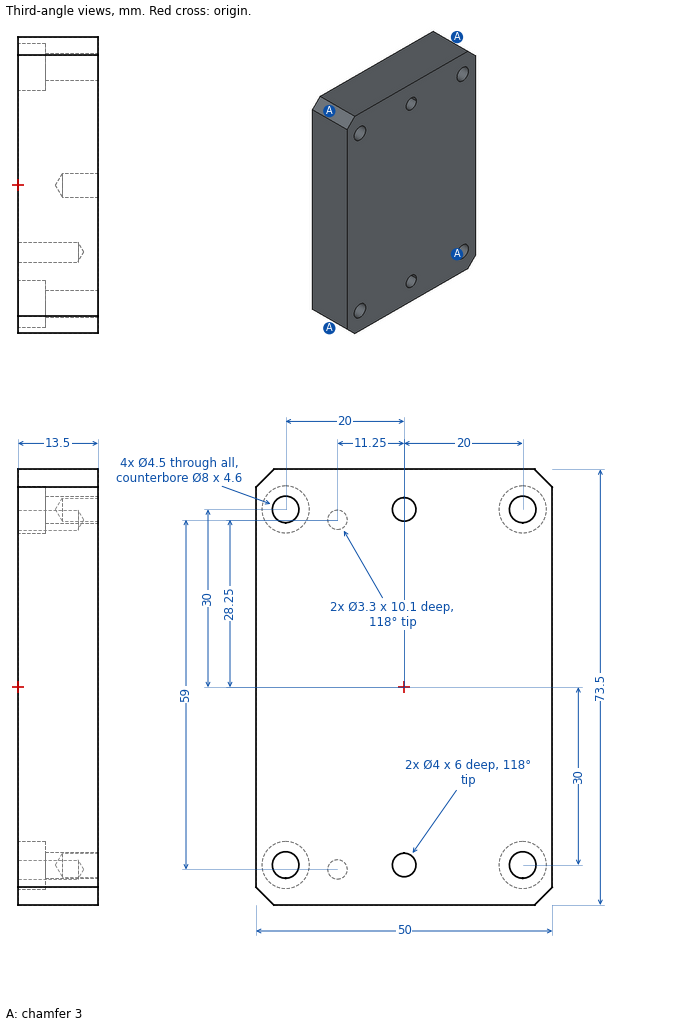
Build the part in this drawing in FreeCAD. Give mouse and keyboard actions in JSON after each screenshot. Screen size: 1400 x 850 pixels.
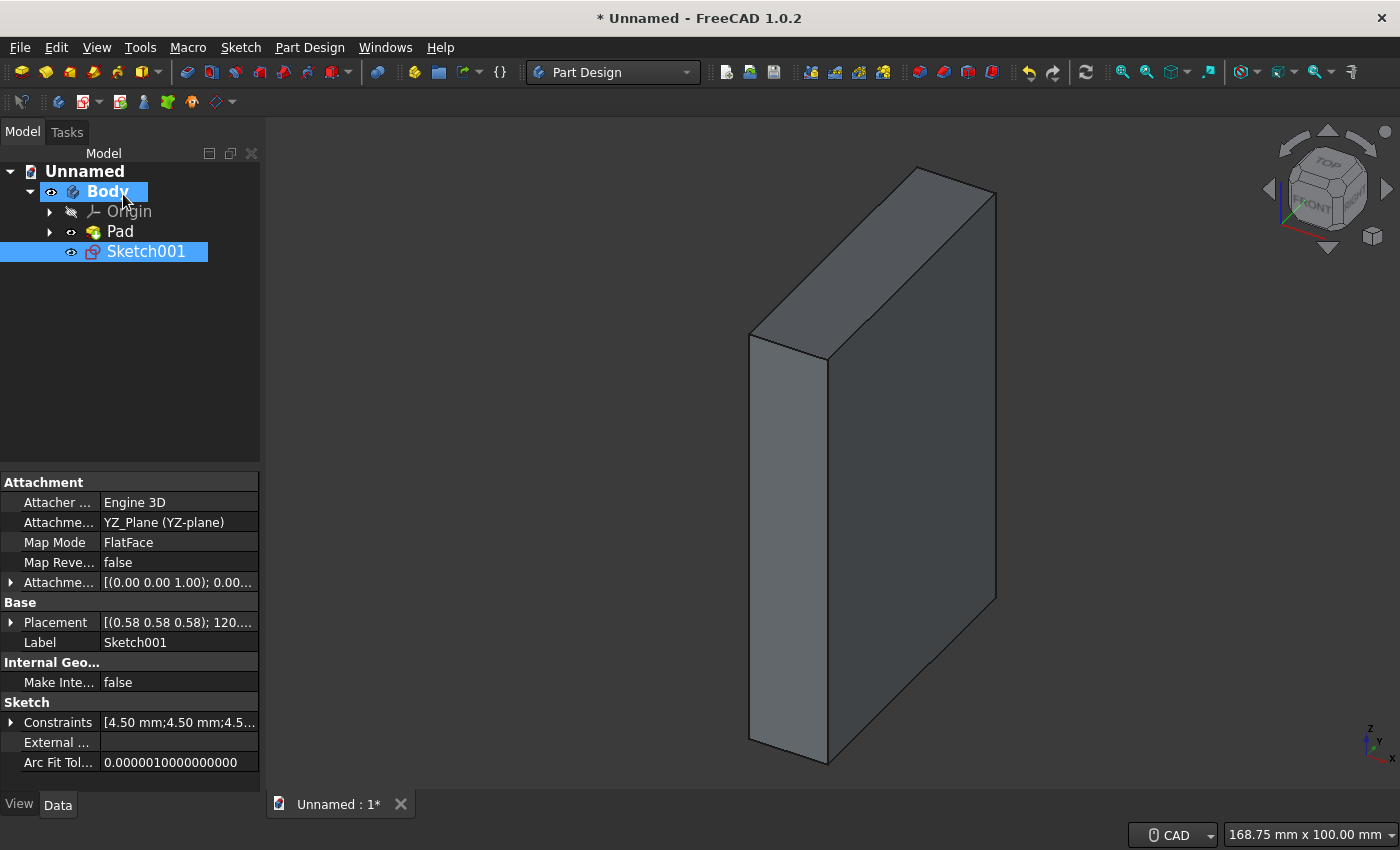
{"action": "left_click", "coordinate": [212, 72]}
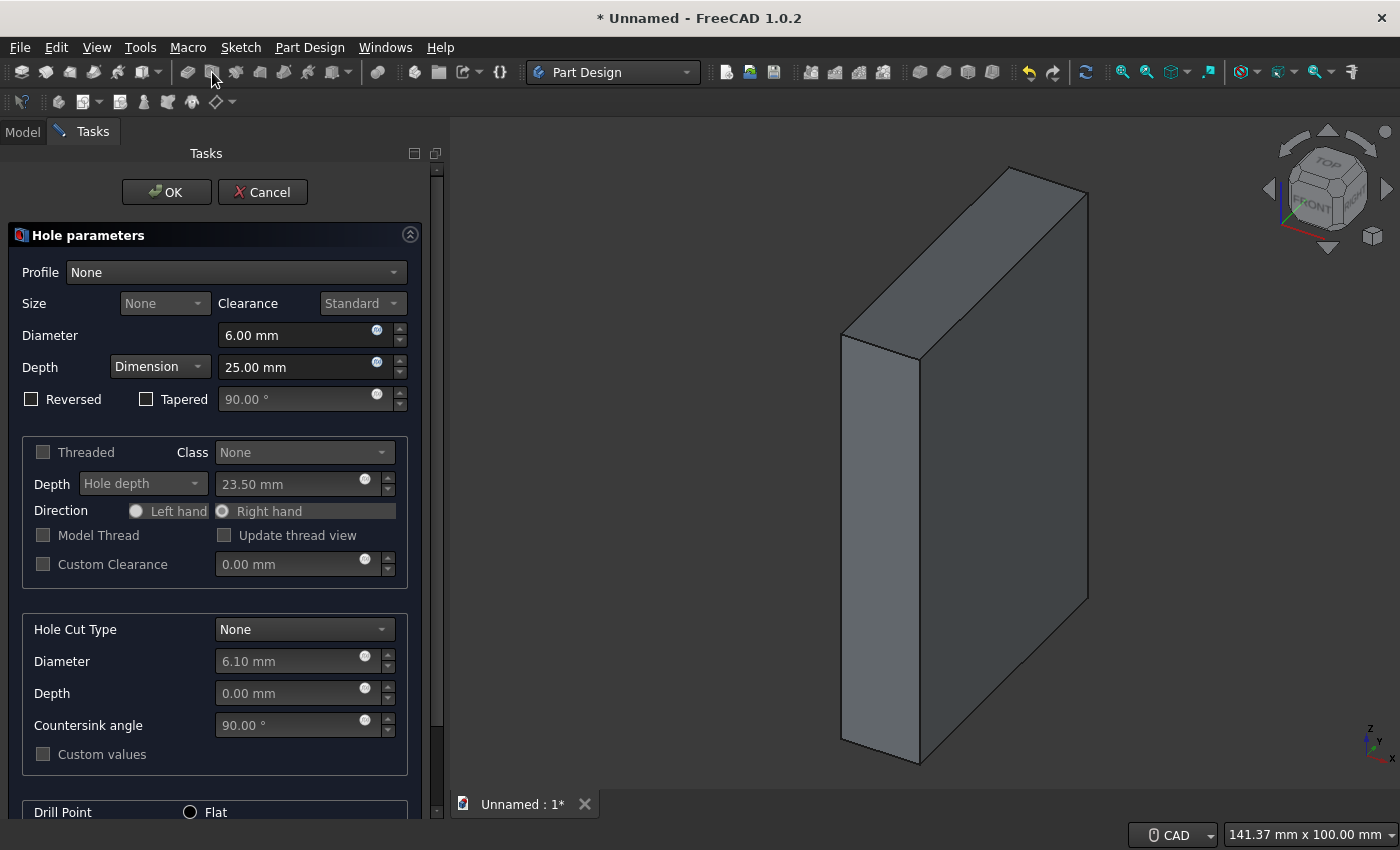
{"action": "triple_click", "coordinate": [305, 335]}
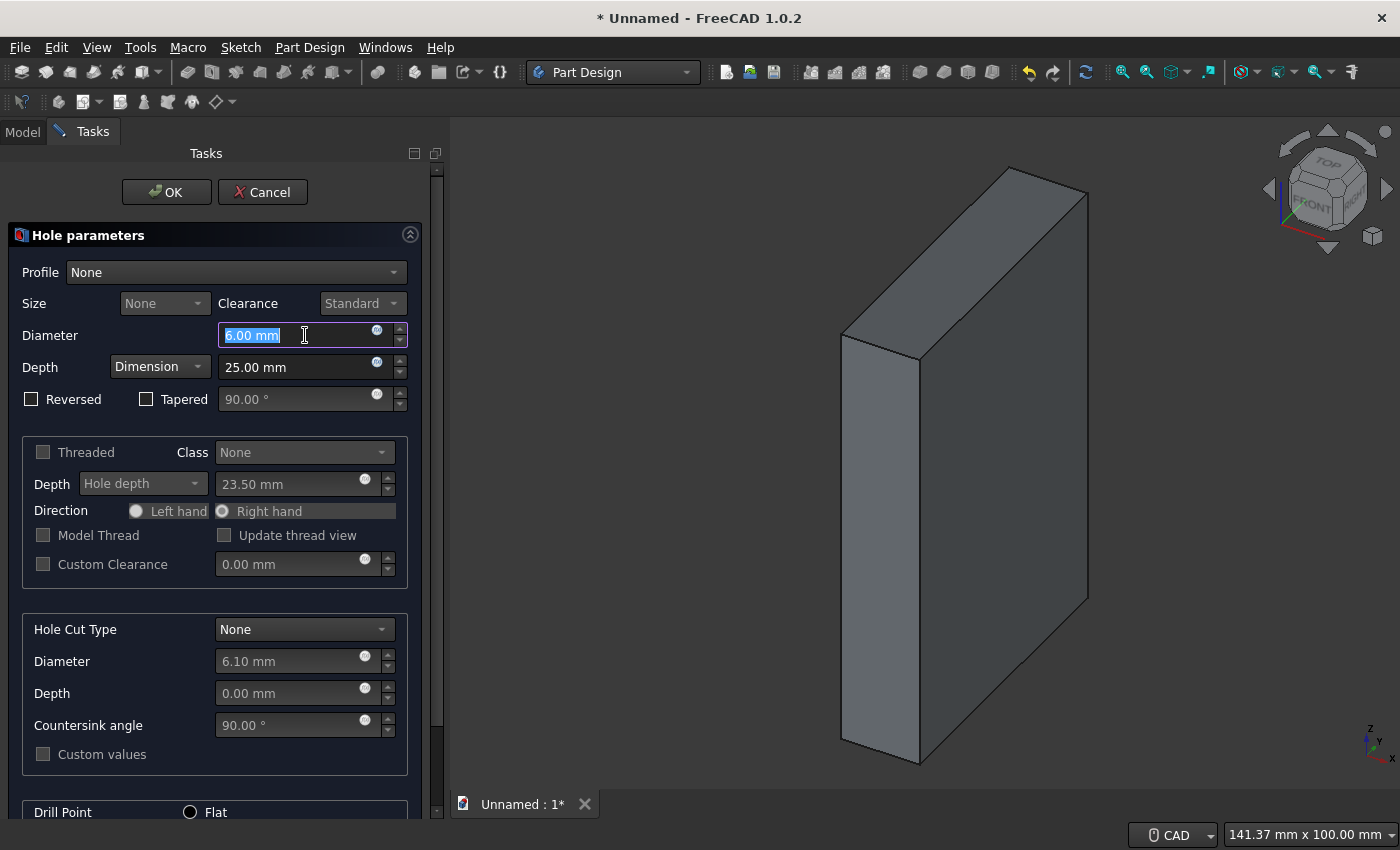
{"action": "type", "text": "4.5"}
{"action": "key", "text": "Tab"}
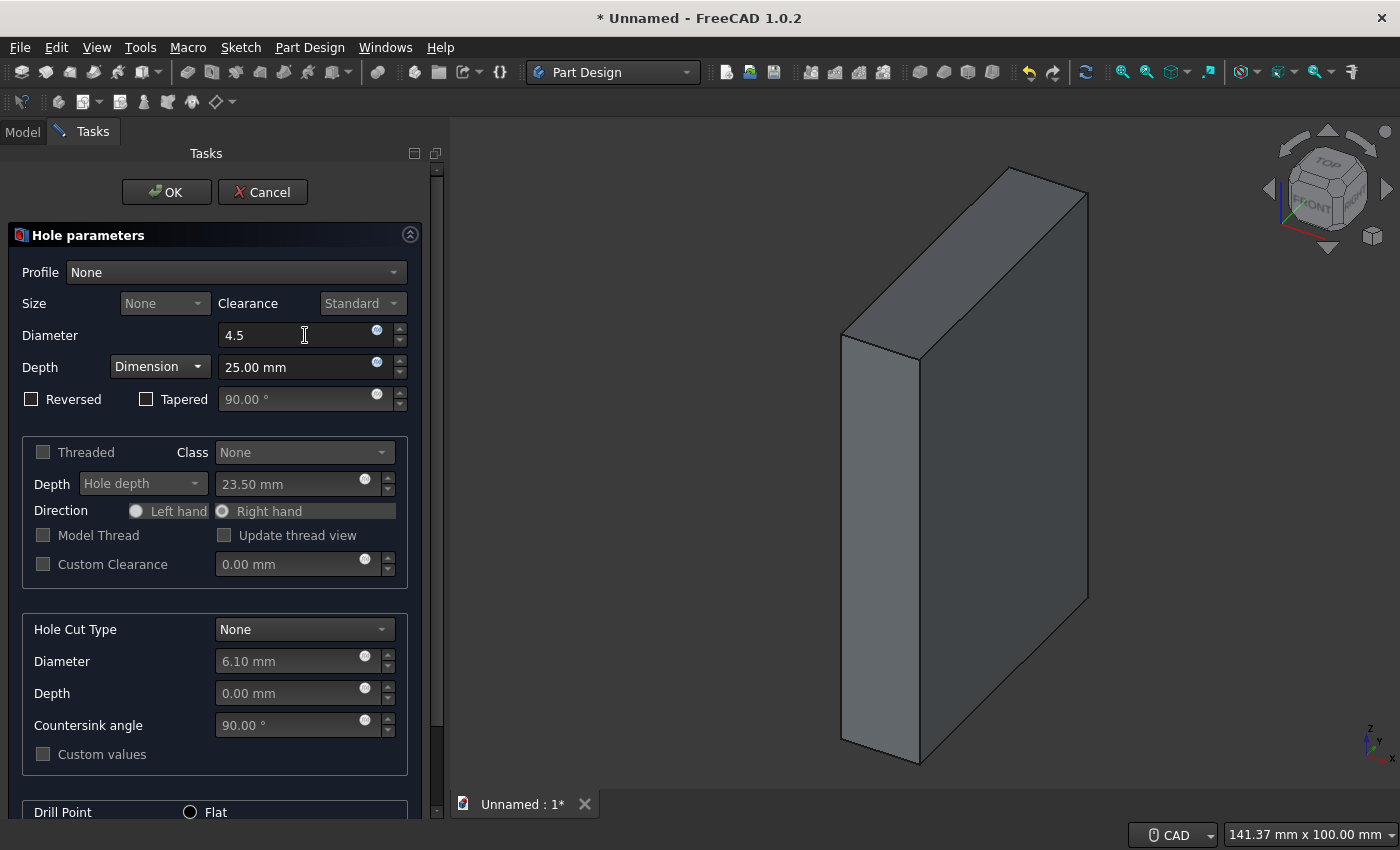
{"action": "left_click", "coordinate": [161, 366]}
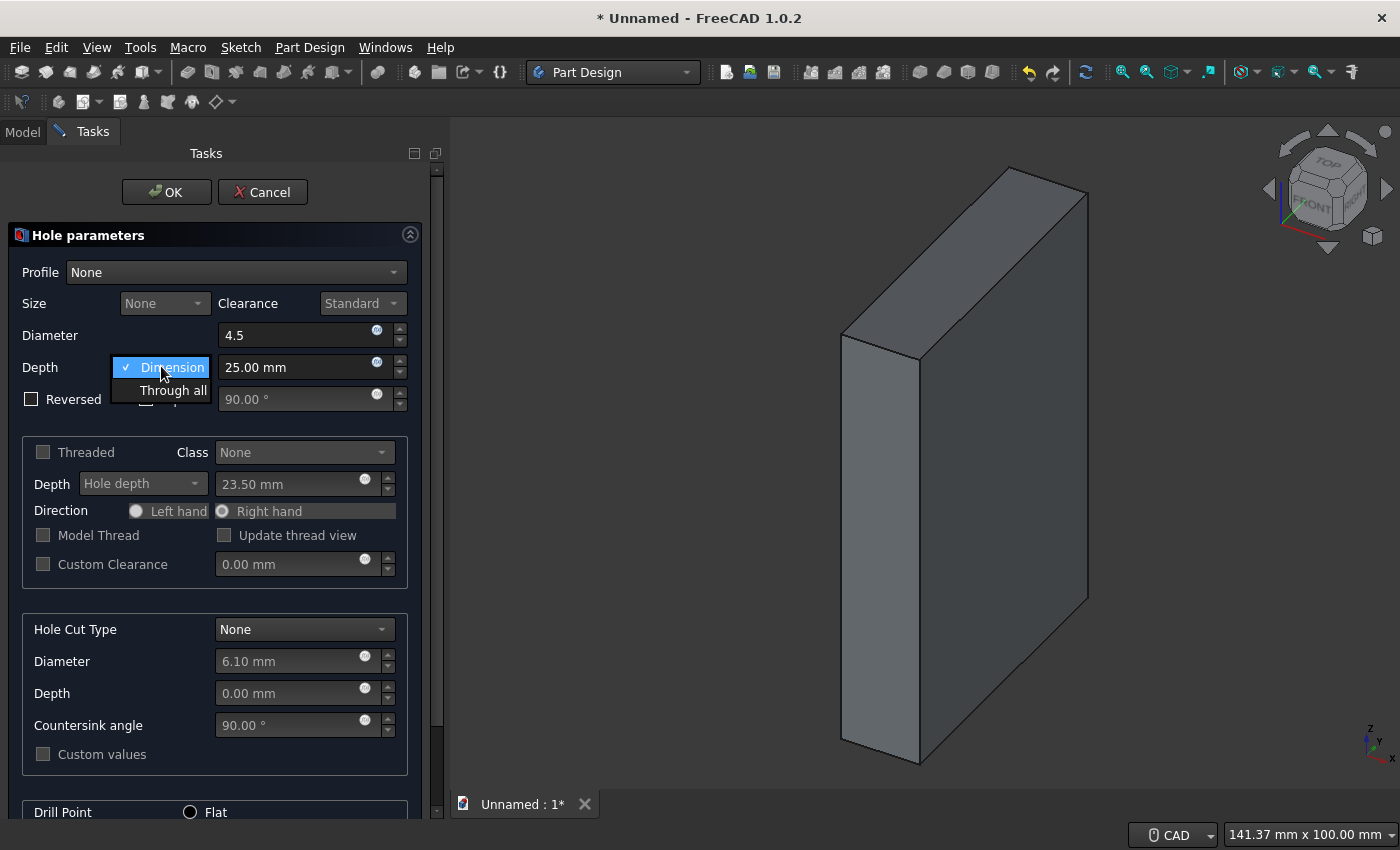
{"action": "left_click", "coordinate": [160, 390]}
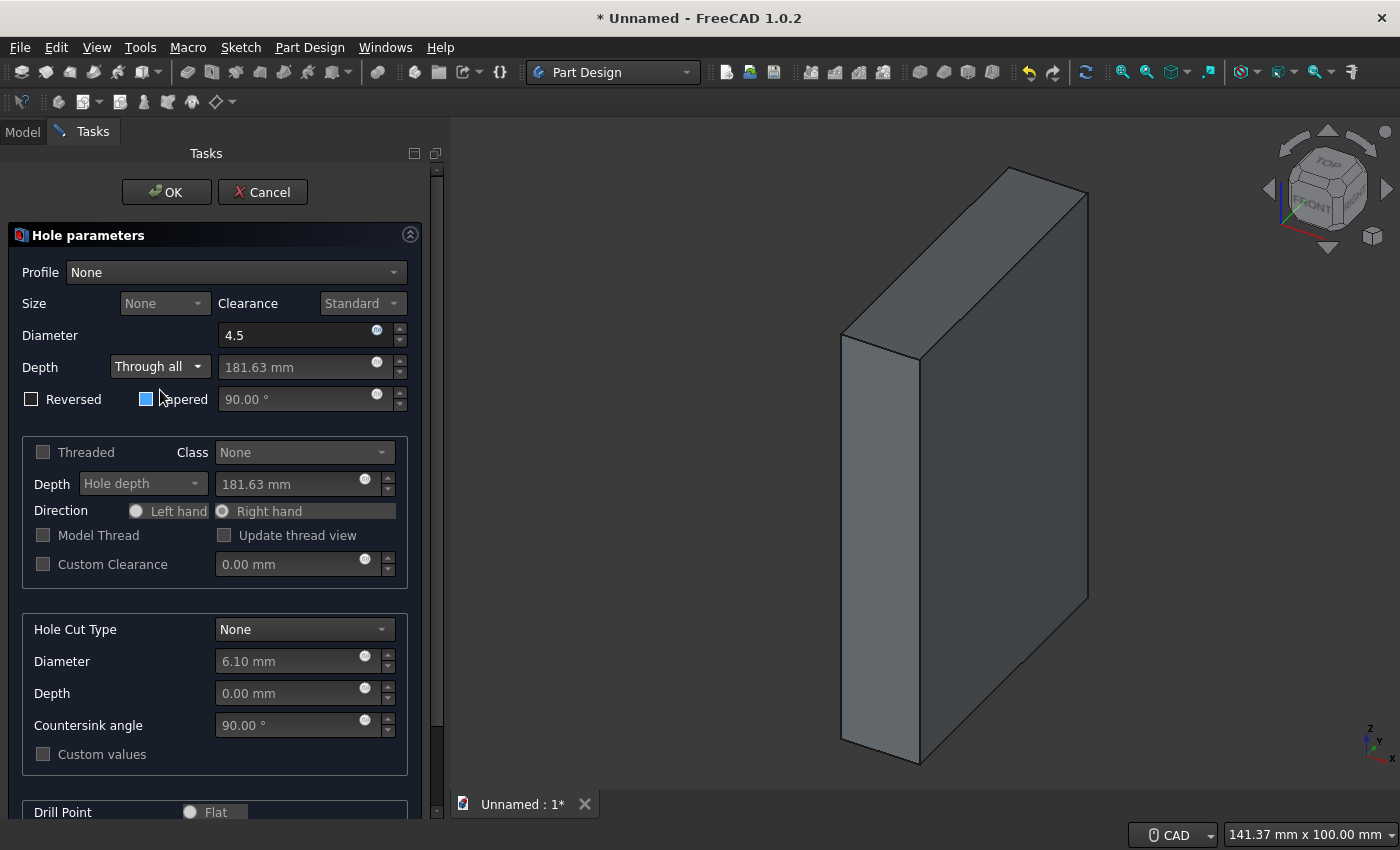
{"action": "left_click", "coordinate": [30, 399]}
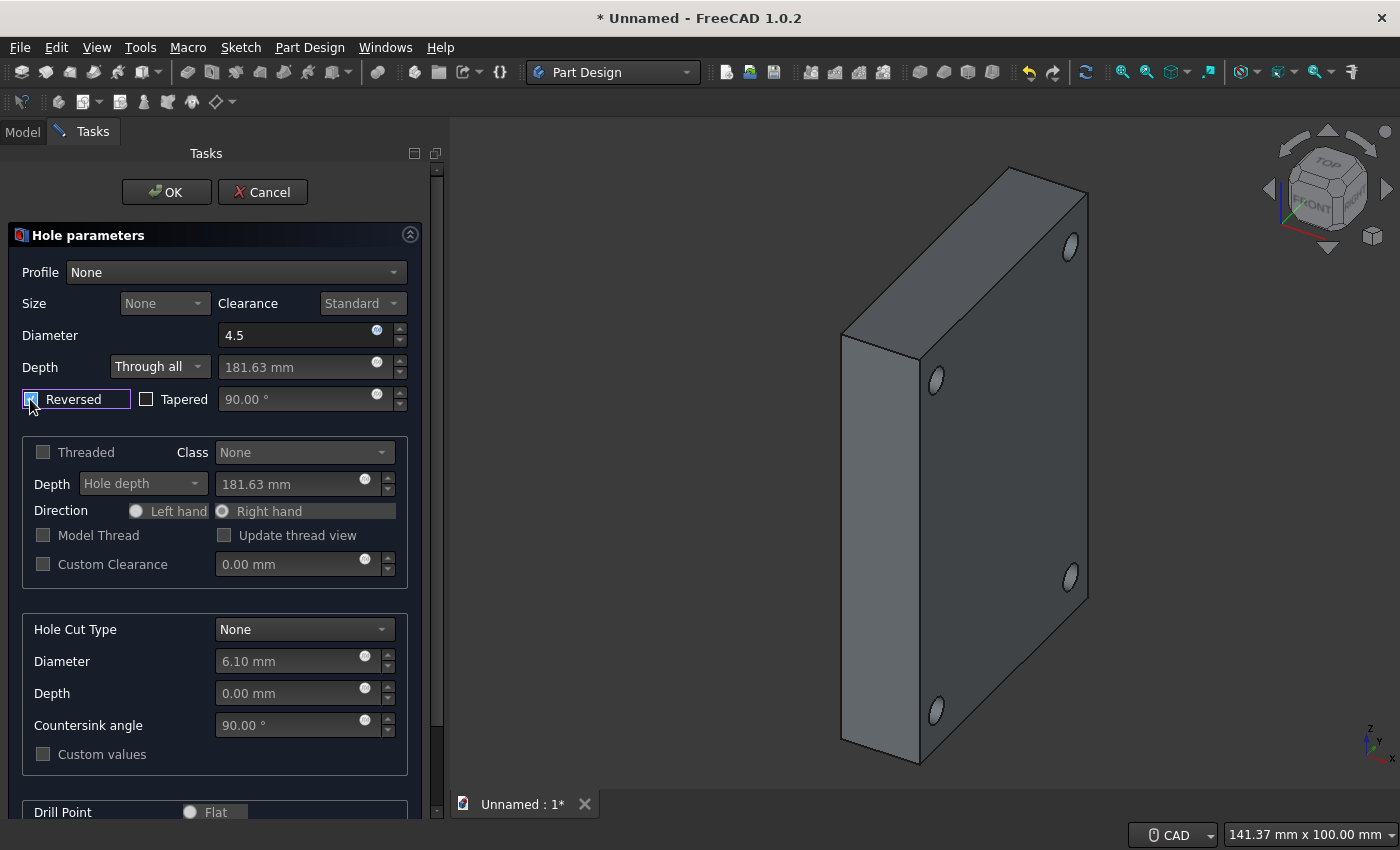
{"action": "left_click", "coordinate": [306, 630]}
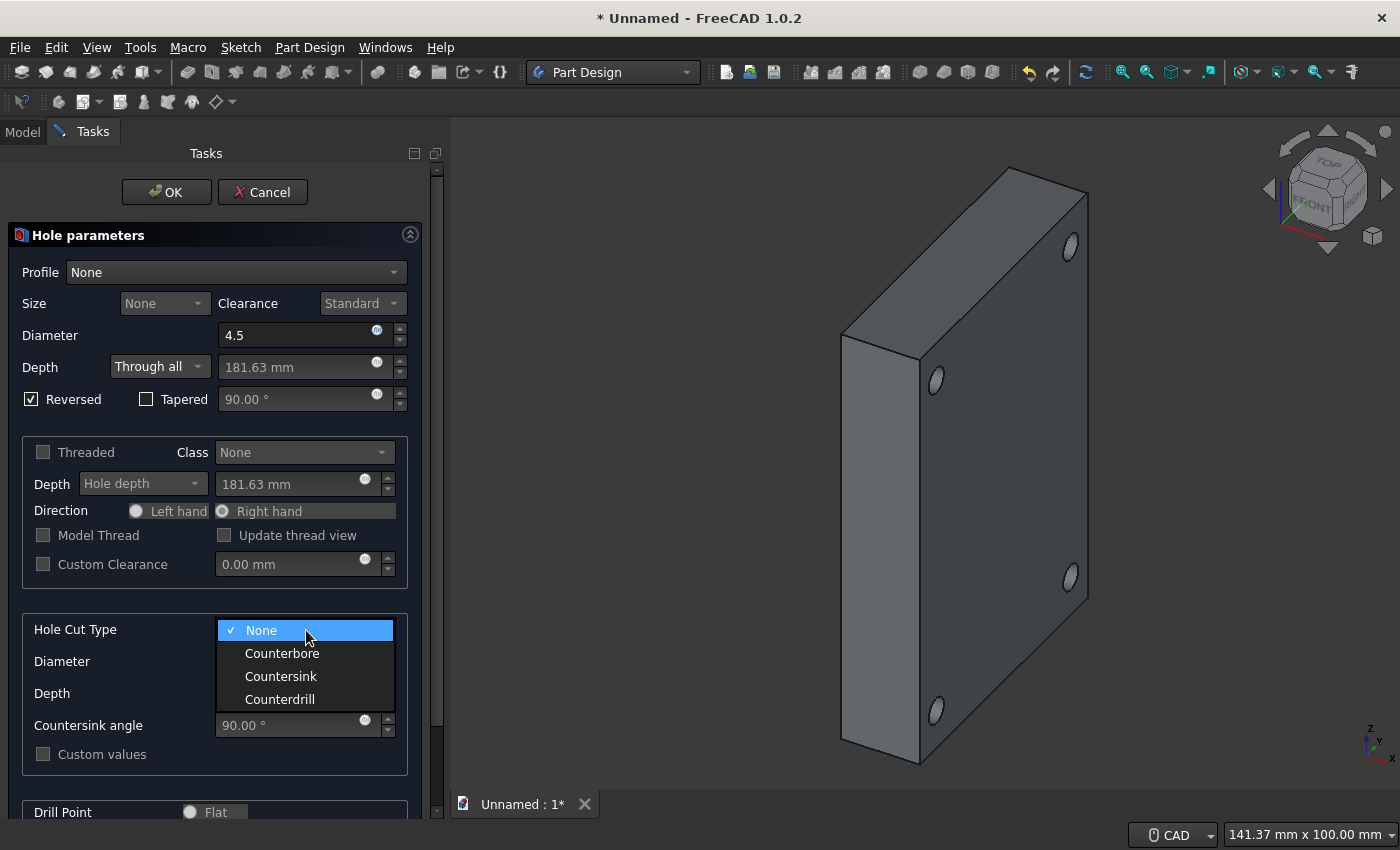
{"action": "left_click", "coordinate": [304, 654]}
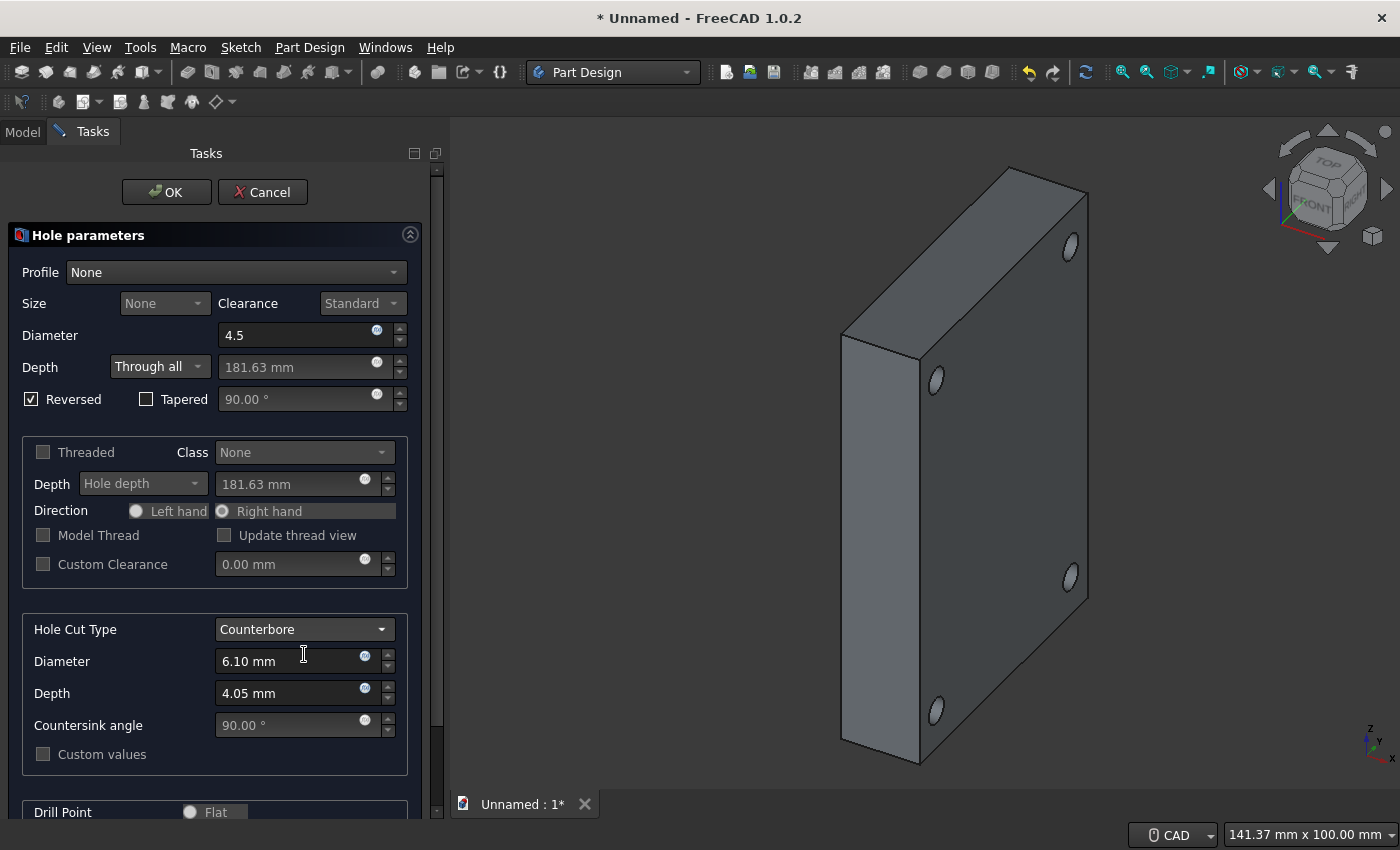
{"action": "triple_click", "coordinate": [298, 661]}